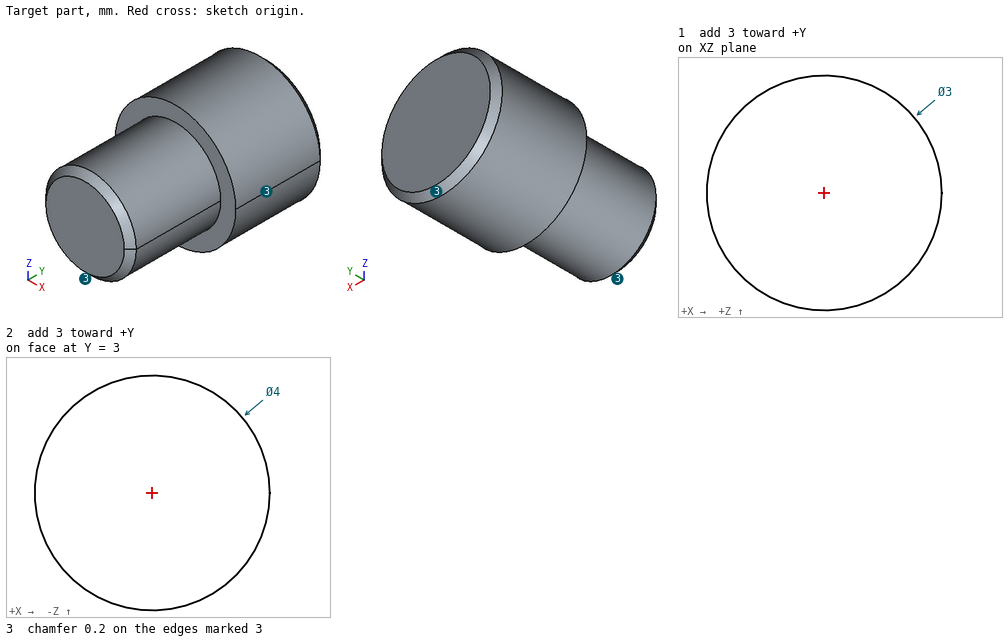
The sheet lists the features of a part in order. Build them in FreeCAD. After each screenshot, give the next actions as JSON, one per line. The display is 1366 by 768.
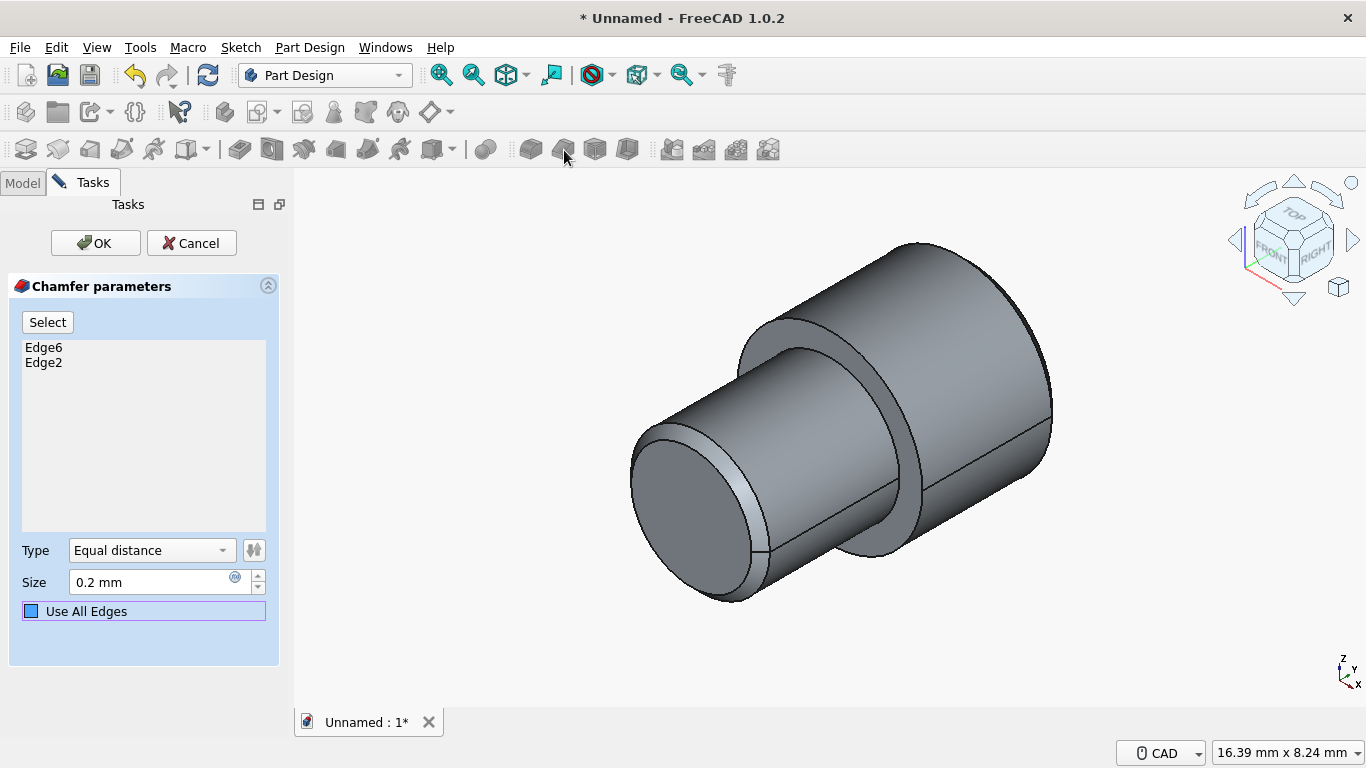
{"action": "left_click", "coordinate": [96, 243]}